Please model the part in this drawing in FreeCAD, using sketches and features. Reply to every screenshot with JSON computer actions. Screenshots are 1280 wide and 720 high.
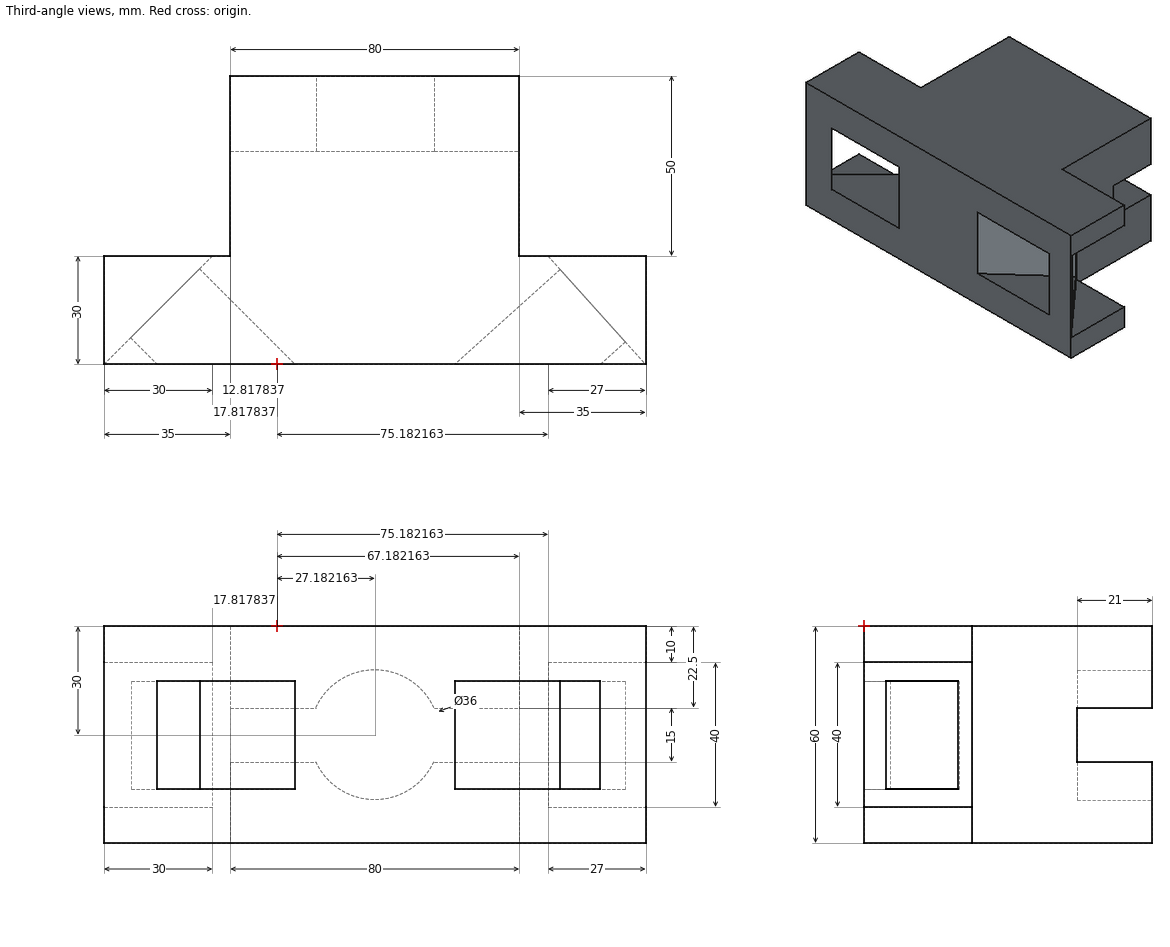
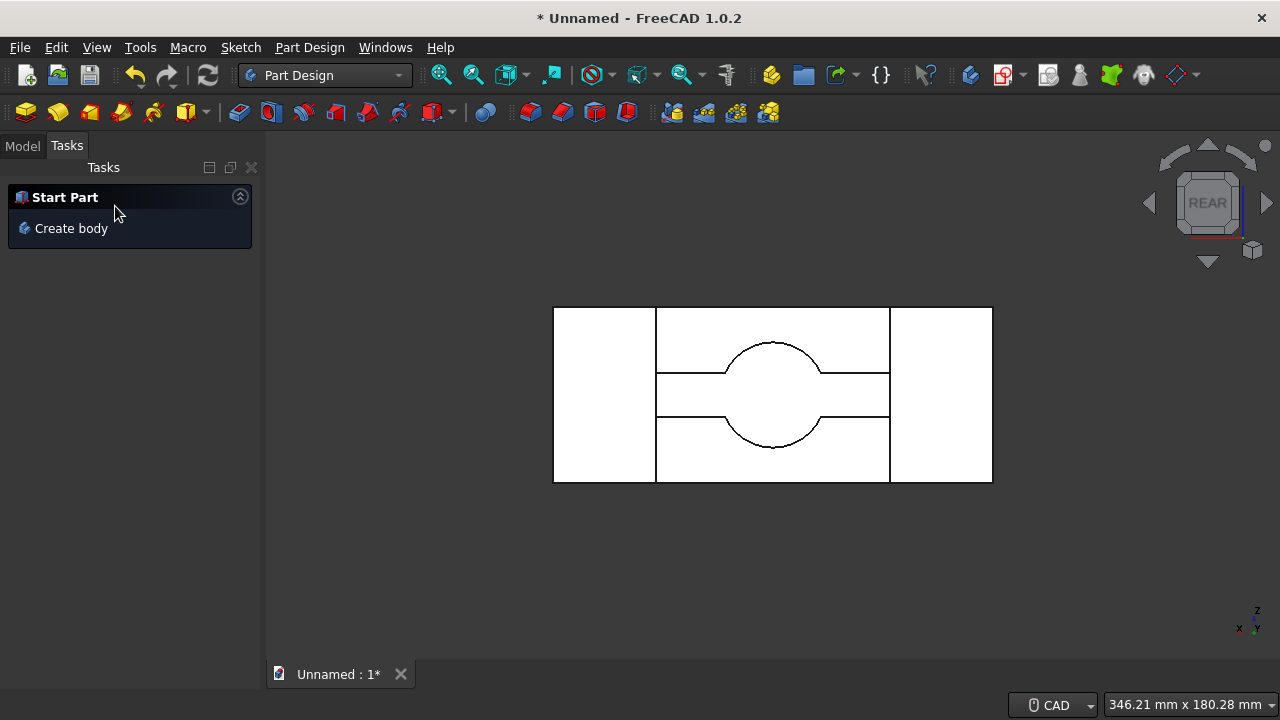
{"action": "left_click", "coordinate": [442, 76]}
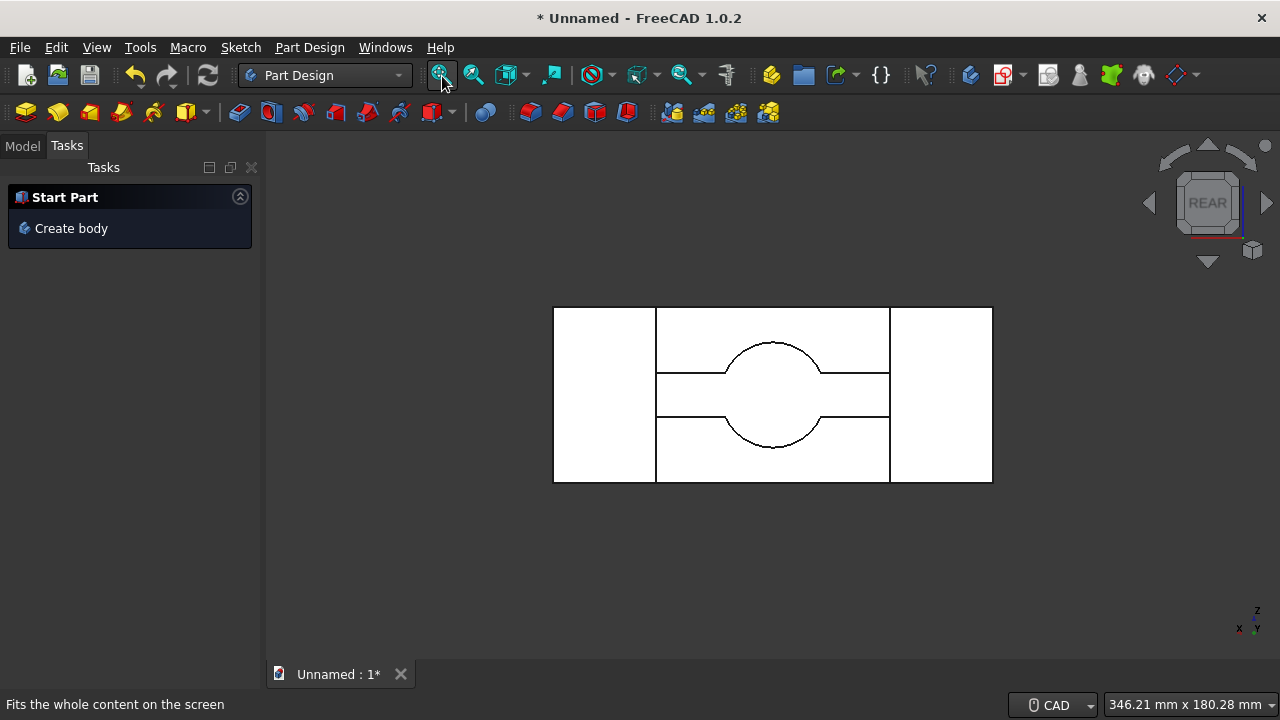
{"action": "left_click", "coordinate": [605, 369]}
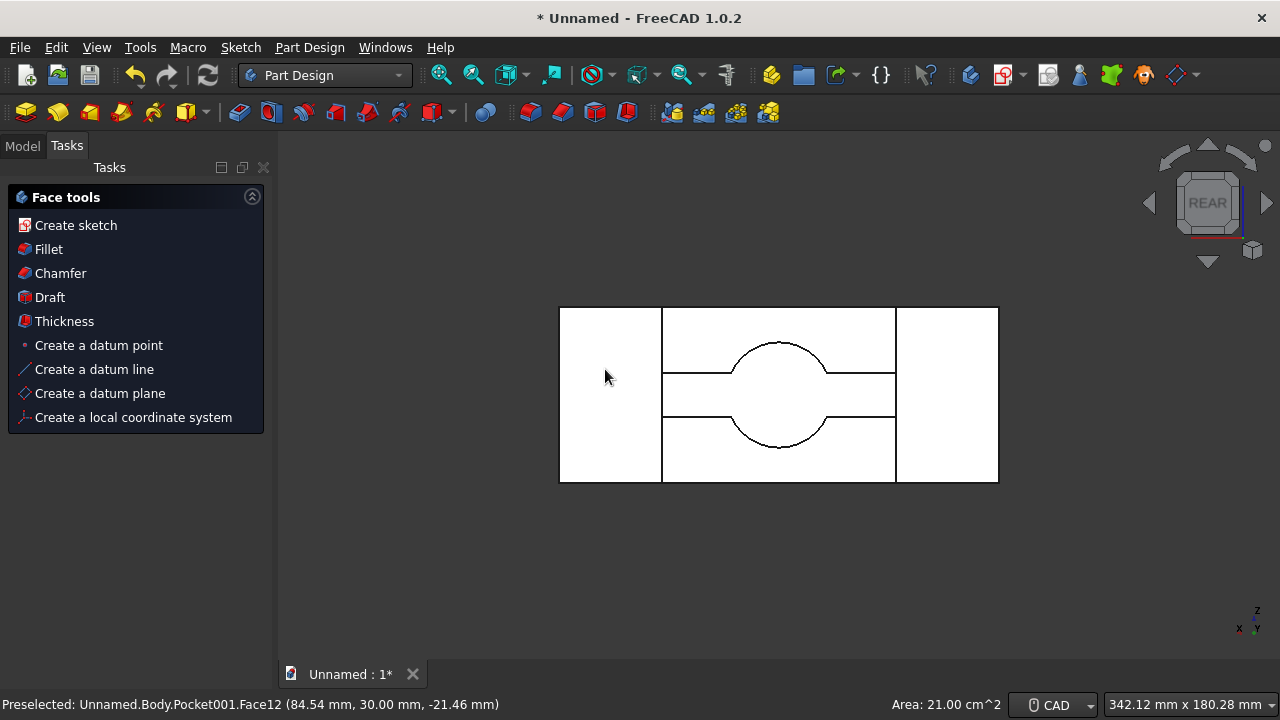
{"action": "left_click", "coordinate": [1004, 76]}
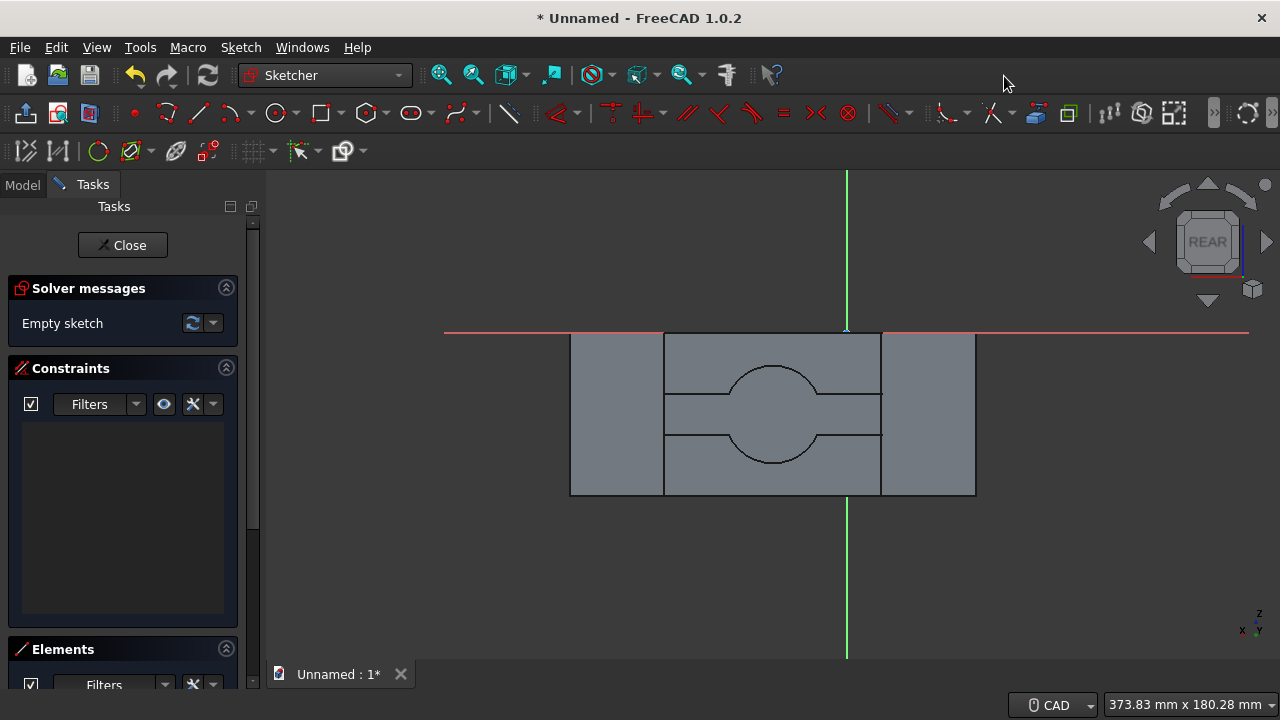
{"action": "scroll", "coordinate": [549, 415], "scroll_direction": "up", "scroll_amount": 5}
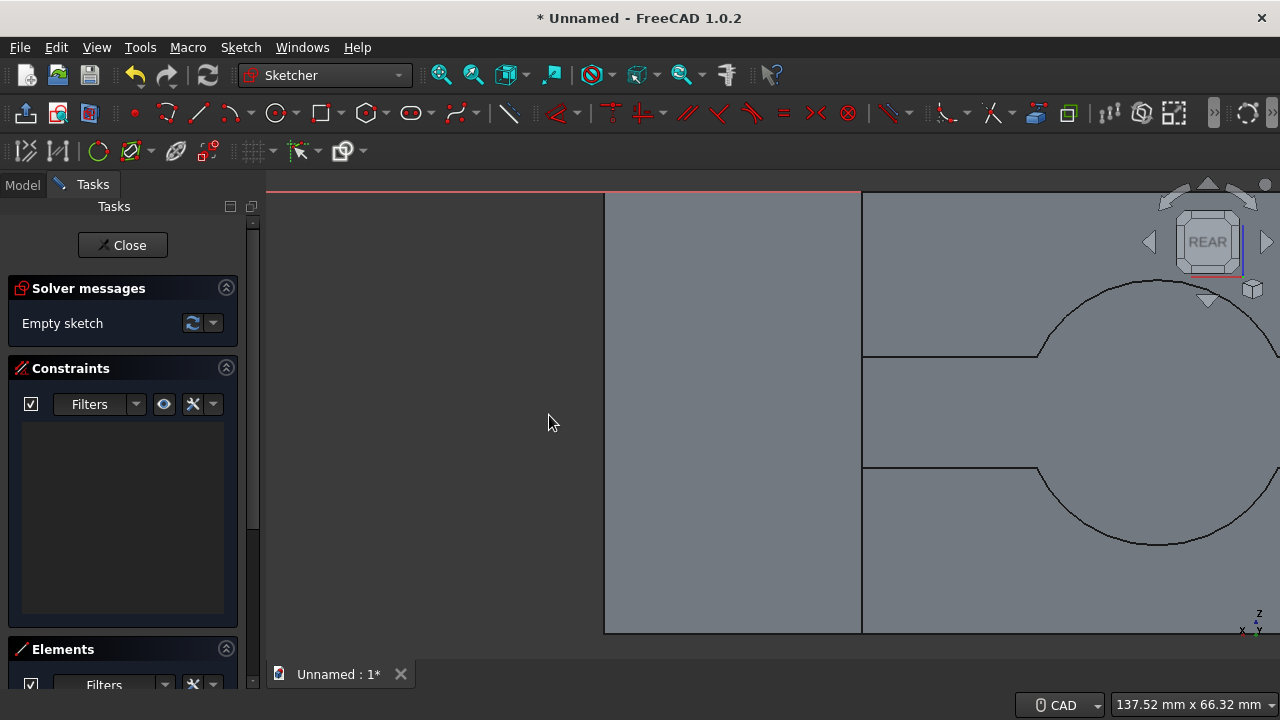
{"action": "left_click", "coordinate": [322, 114]}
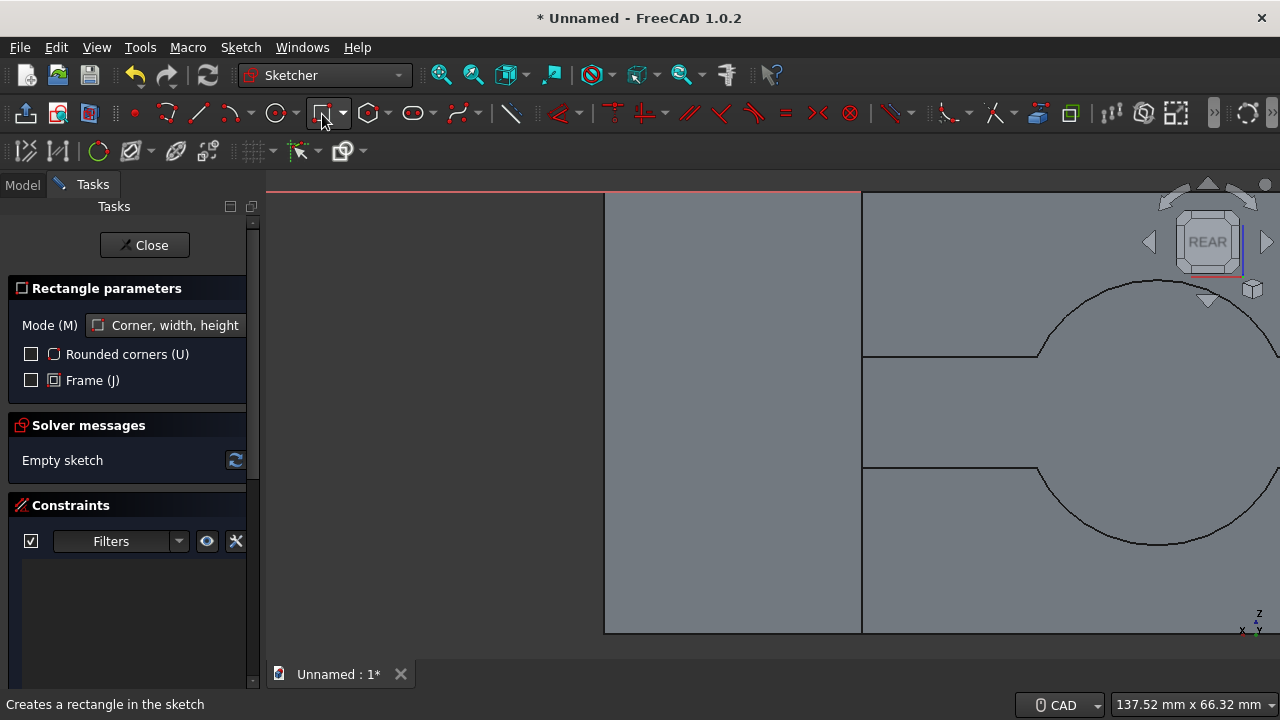
{"action": "left_click", "coordinate": [604, 265]}
{"action": "left_click", "coordinate": [803, 560]}
{"action": "key", "text": "Escape"}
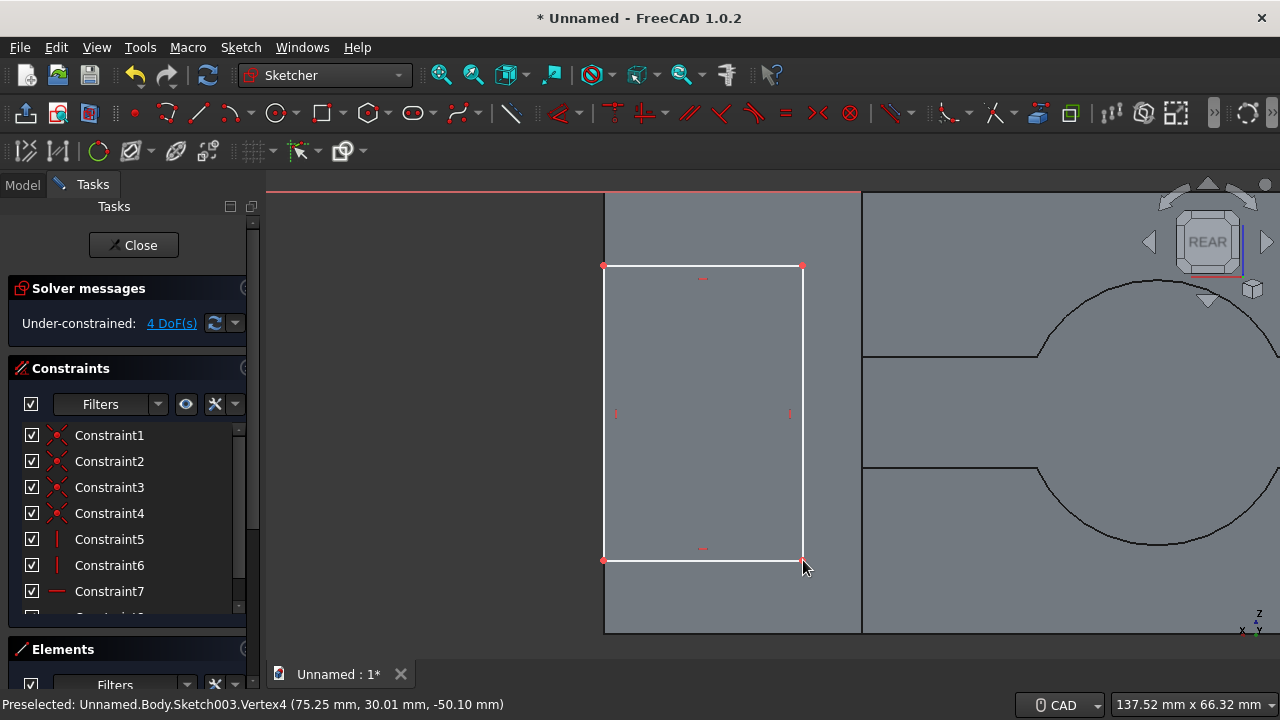
{"action": "left_click", "coordinate": [558, 114]}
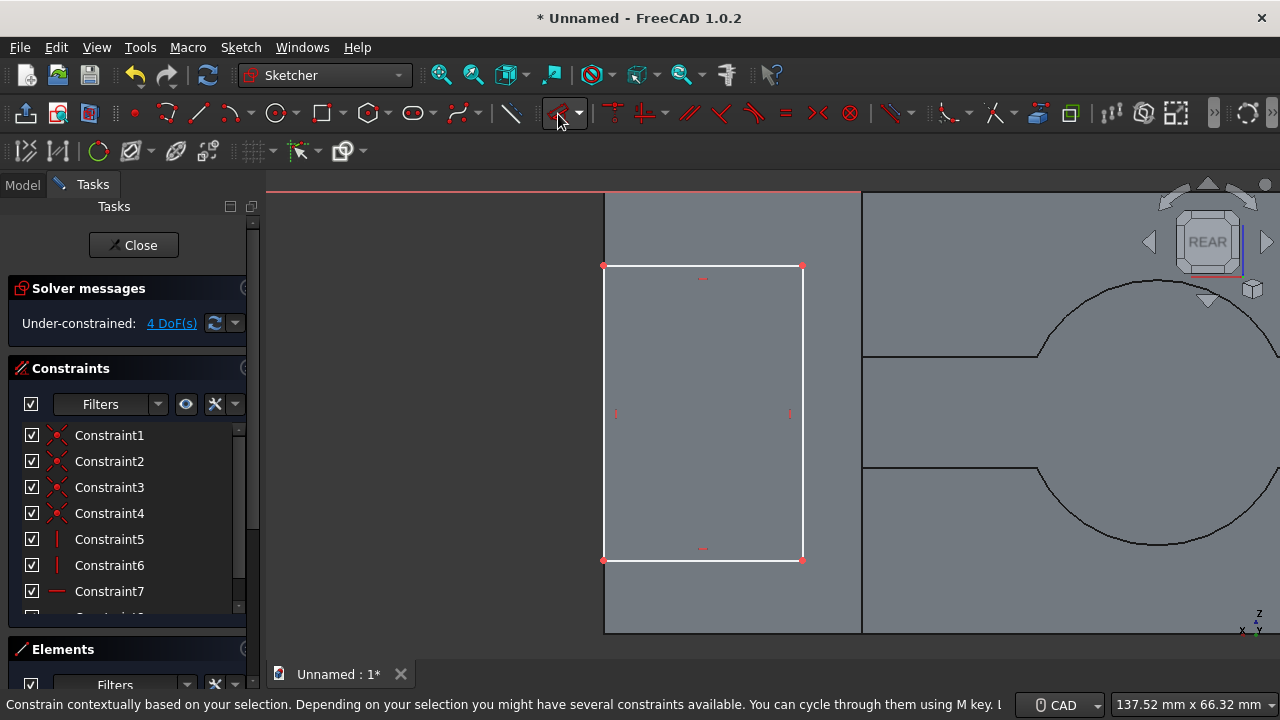
{"action": "left_click", "coordinate": [604, 355]}
{"action": "left_click", "coordinate": [570, 414]}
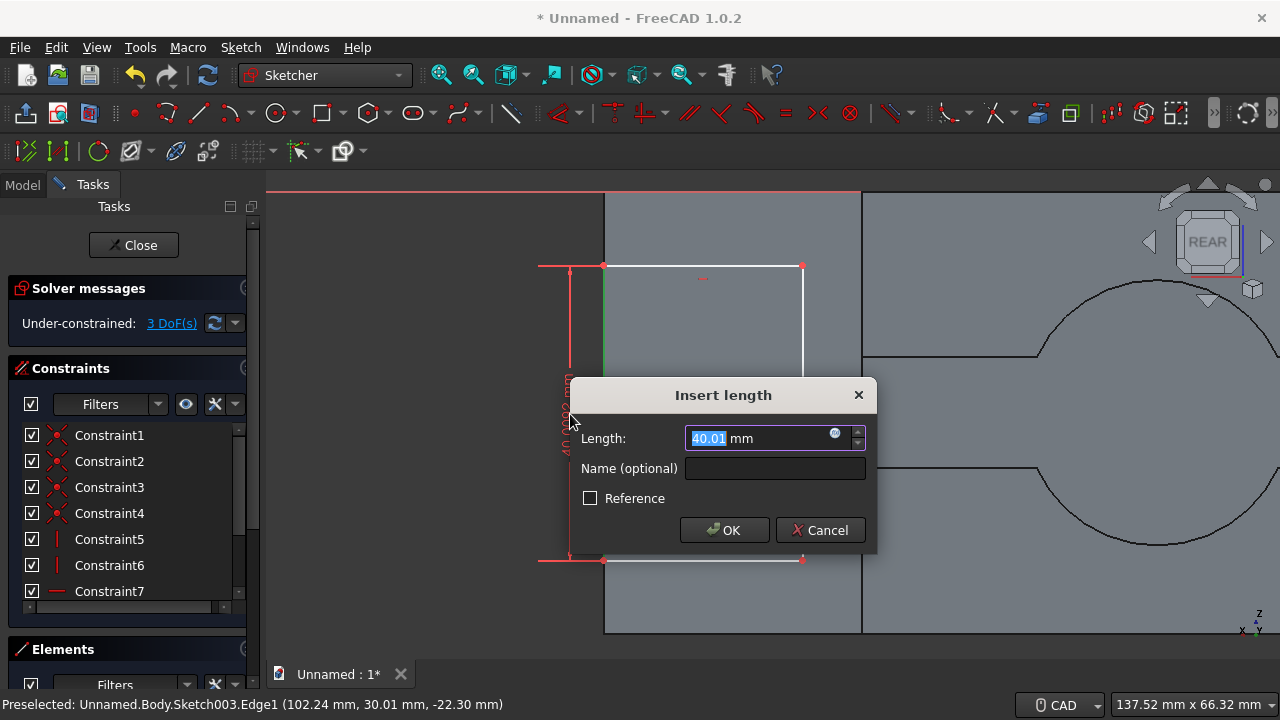
{"action": "type", "text": "40"}
{"action": "key", "text": "Return"}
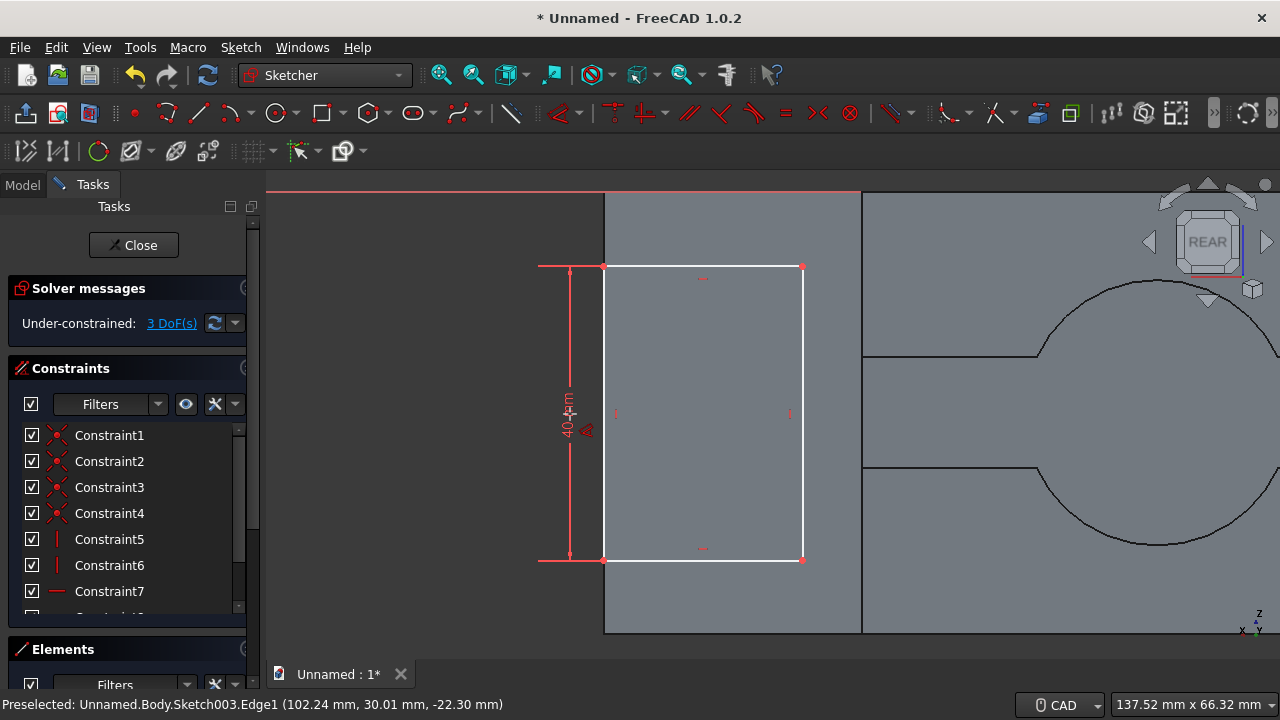
{"action": "left_click", "coordinate": [664, 561]}
{"action": "left_click", "coordinate": [703, 595]}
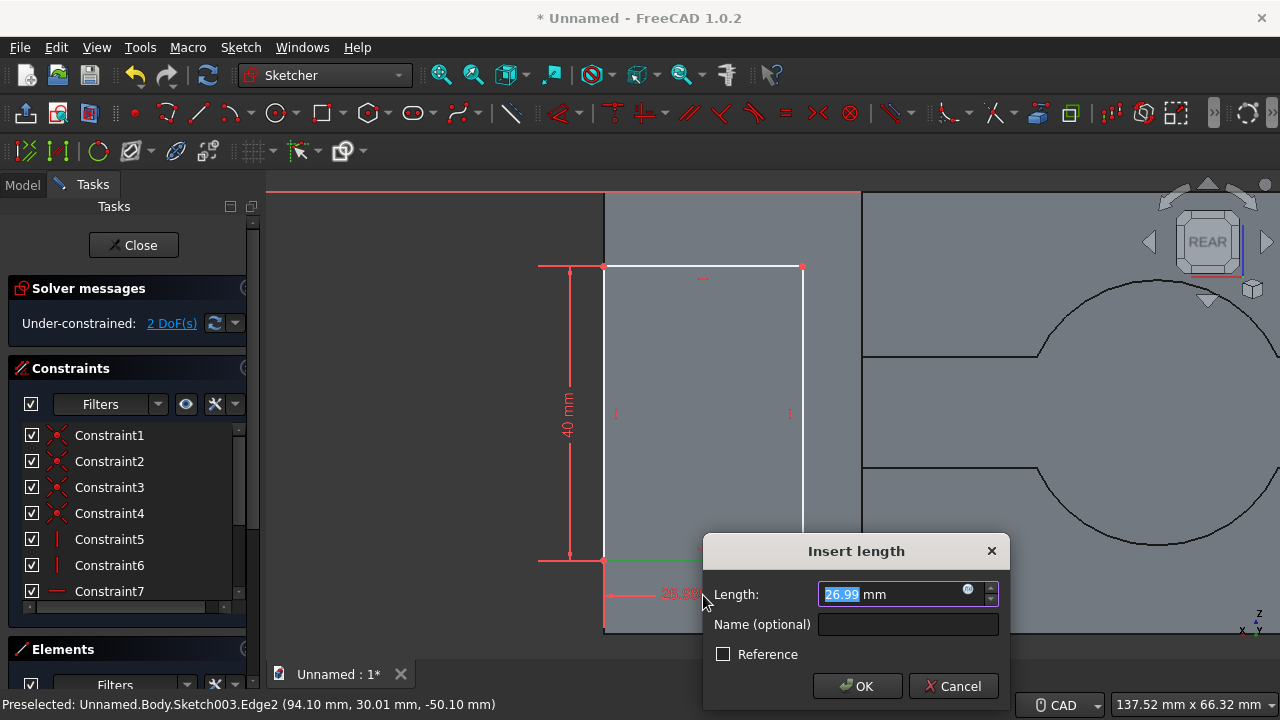
{"action": "type", "text": "27"}
{"action": "key", "text": "Return"}